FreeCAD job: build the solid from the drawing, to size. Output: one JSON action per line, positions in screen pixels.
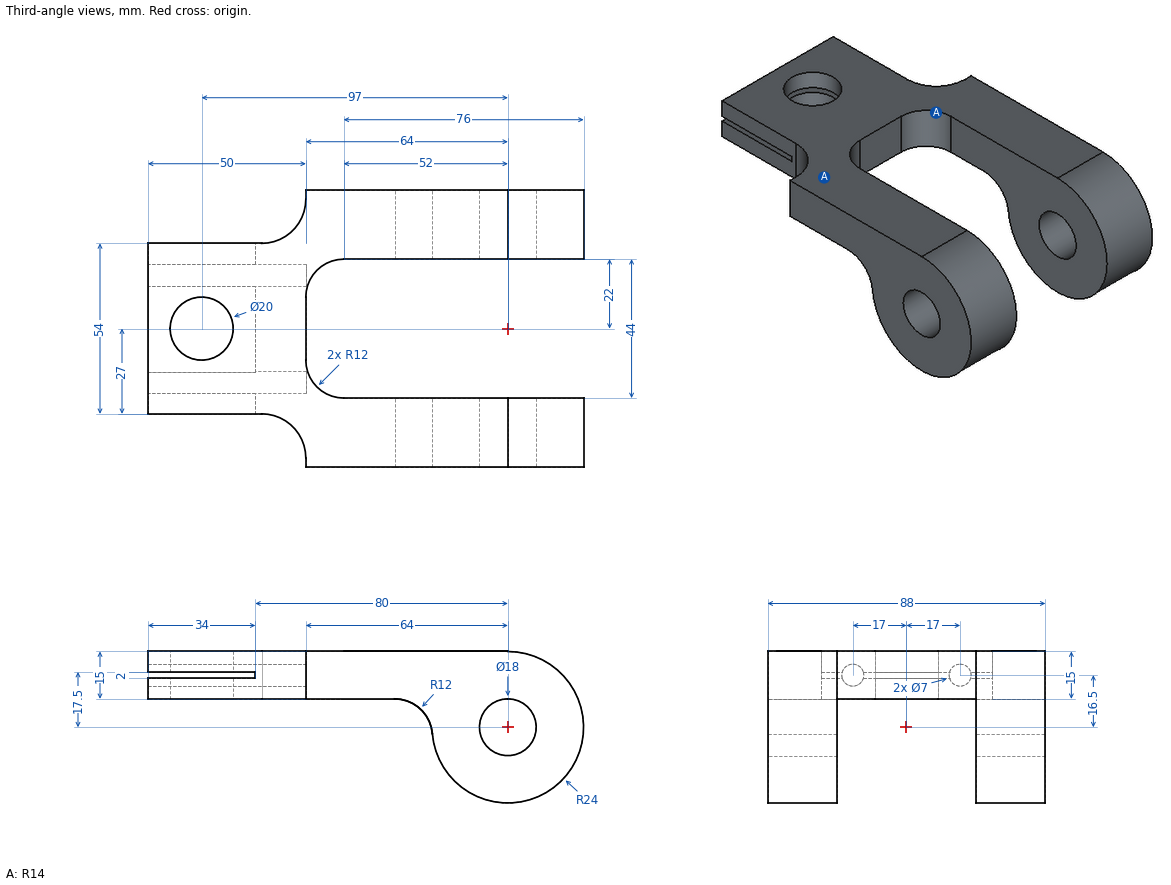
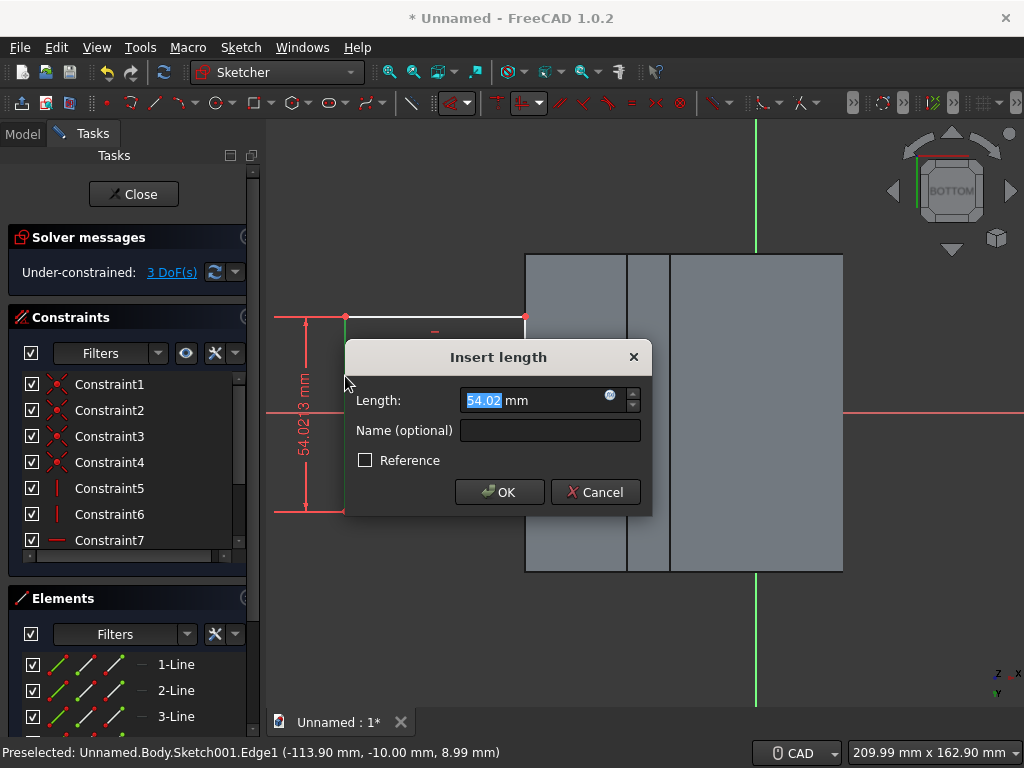
{"action": "type", "text": "54"}
{"action": "key", "text": "Return"}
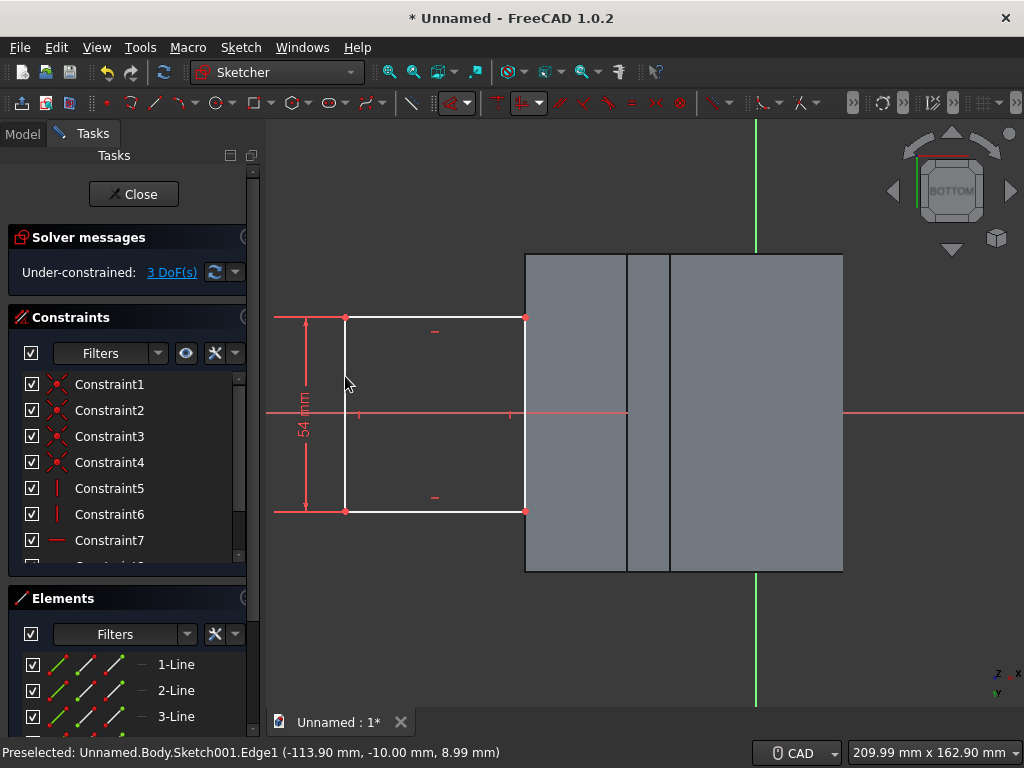
{"action": "left_click", "coordinate": [399, 512]}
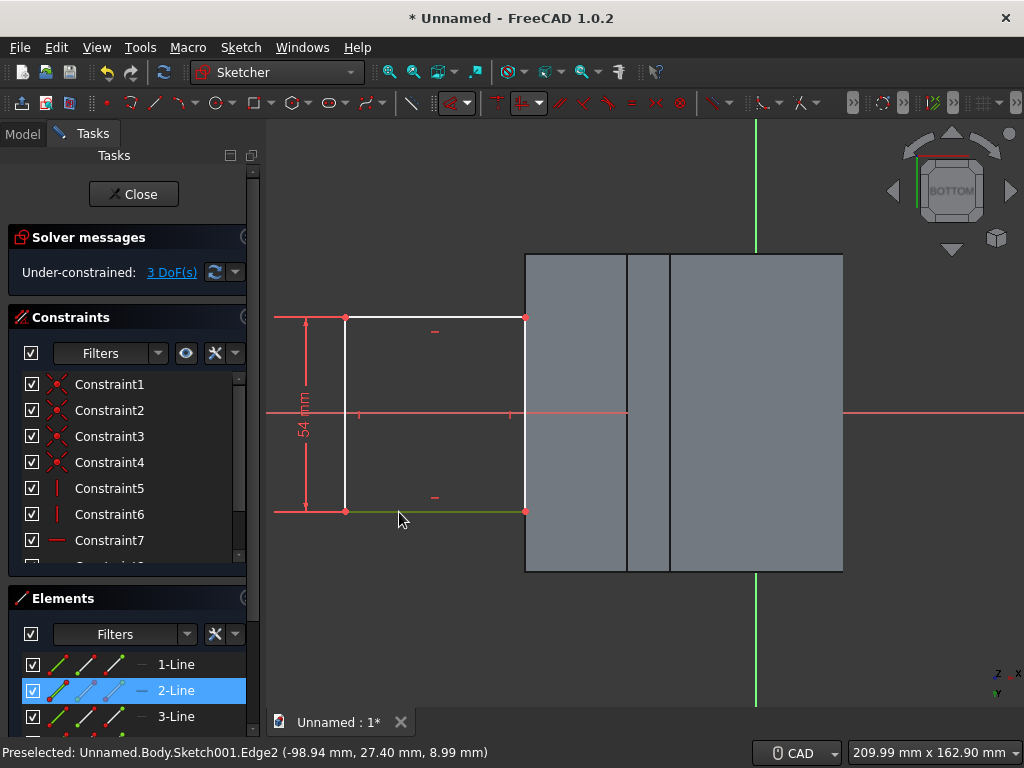
{"action": "key", "text": "l"}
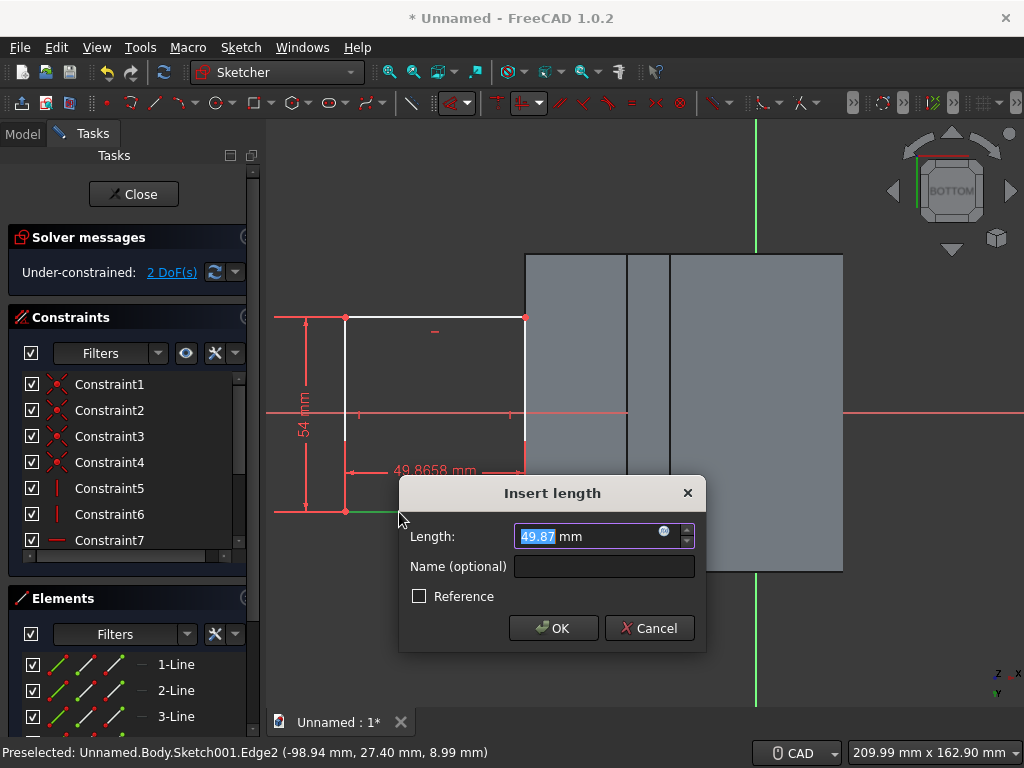
{"action": "type", "text": "50"}
{"action": "key", "text": "Return"}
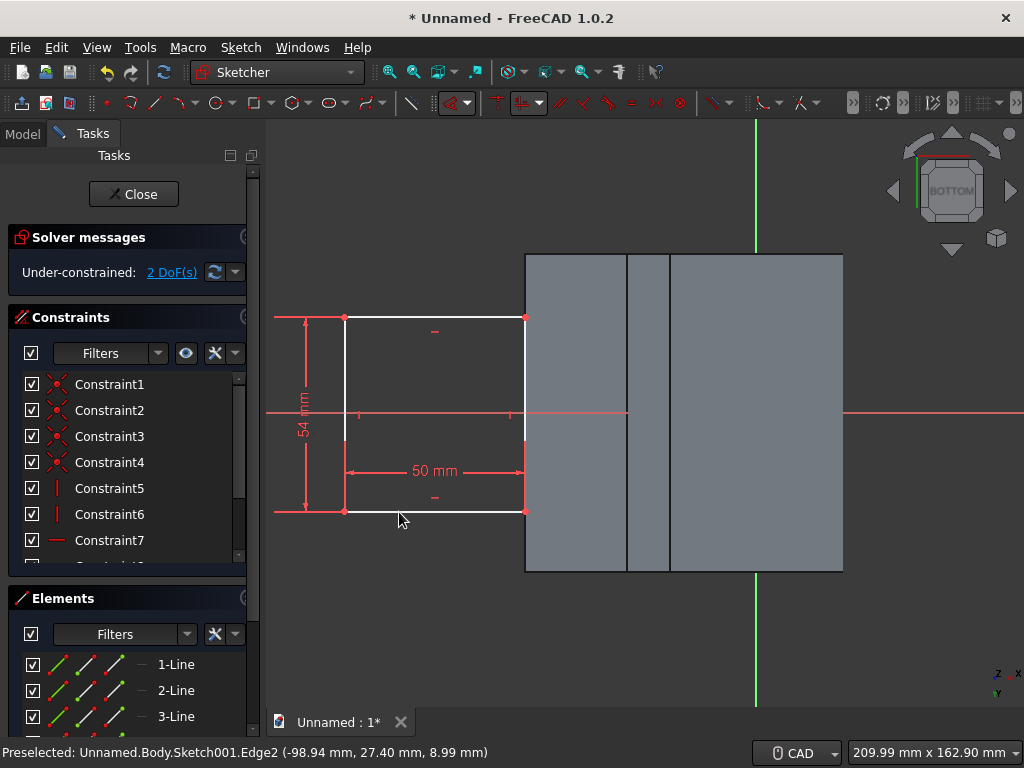
{"action": "left_click", "coordinate": [345, 317]}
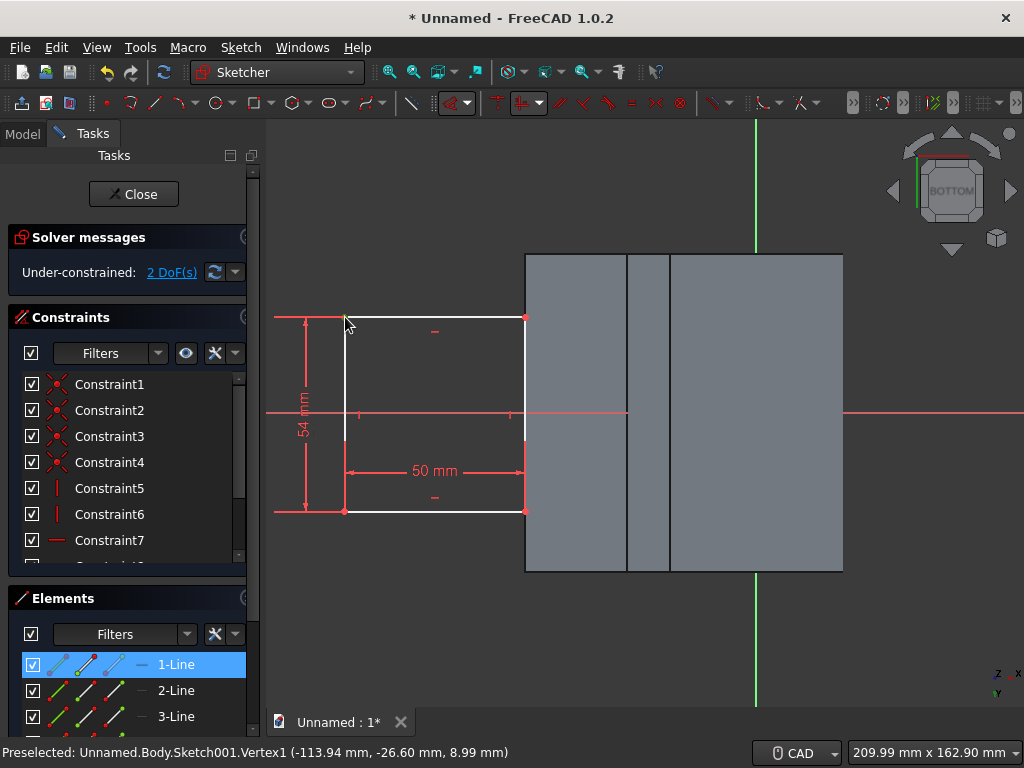
{"action": "key", "text": "i"}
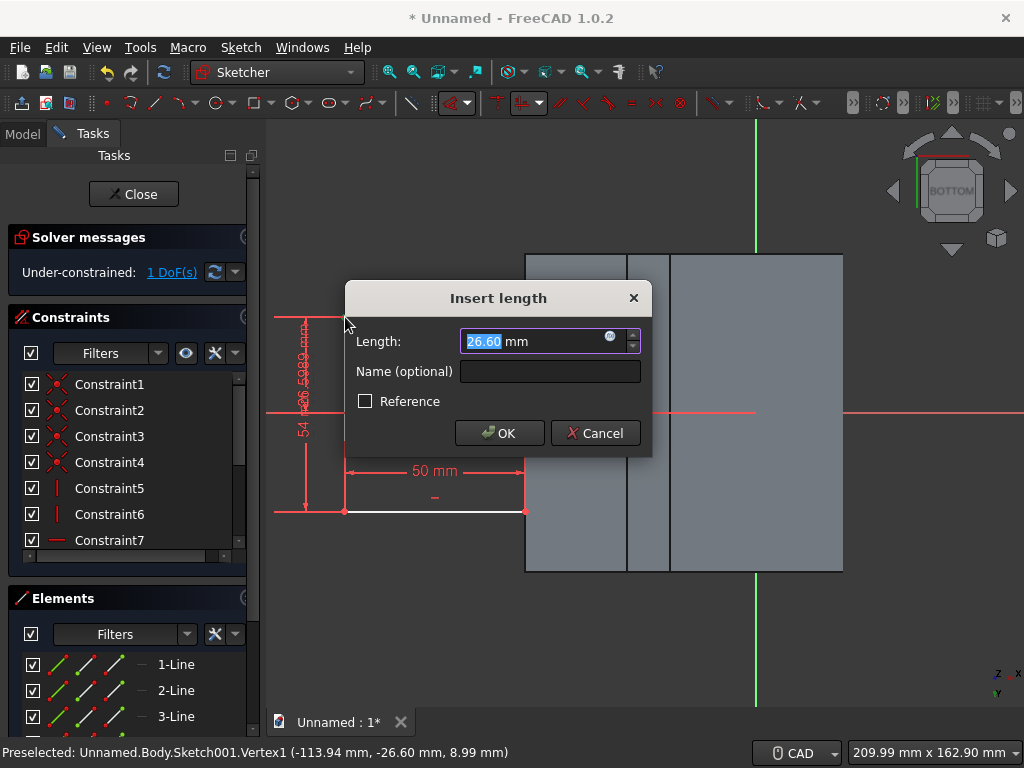
{"action": "type", "text": "27"}
{"action": "key", "text": "Return"}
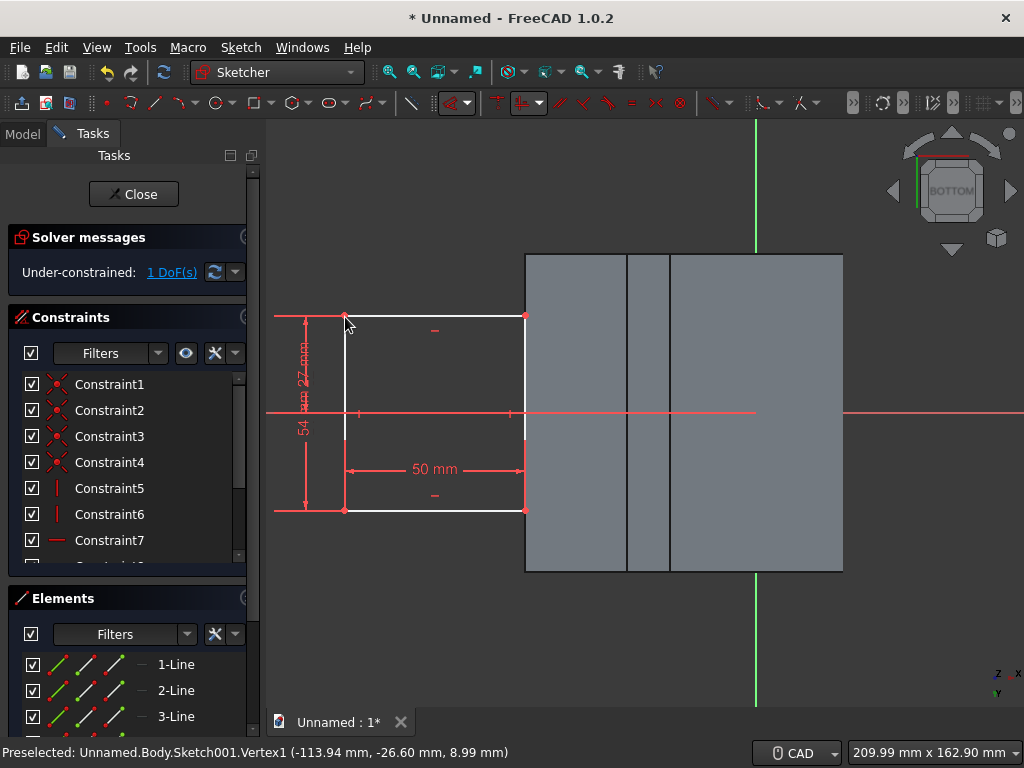
{"action": "left_click", "coordinate": [525, 511]}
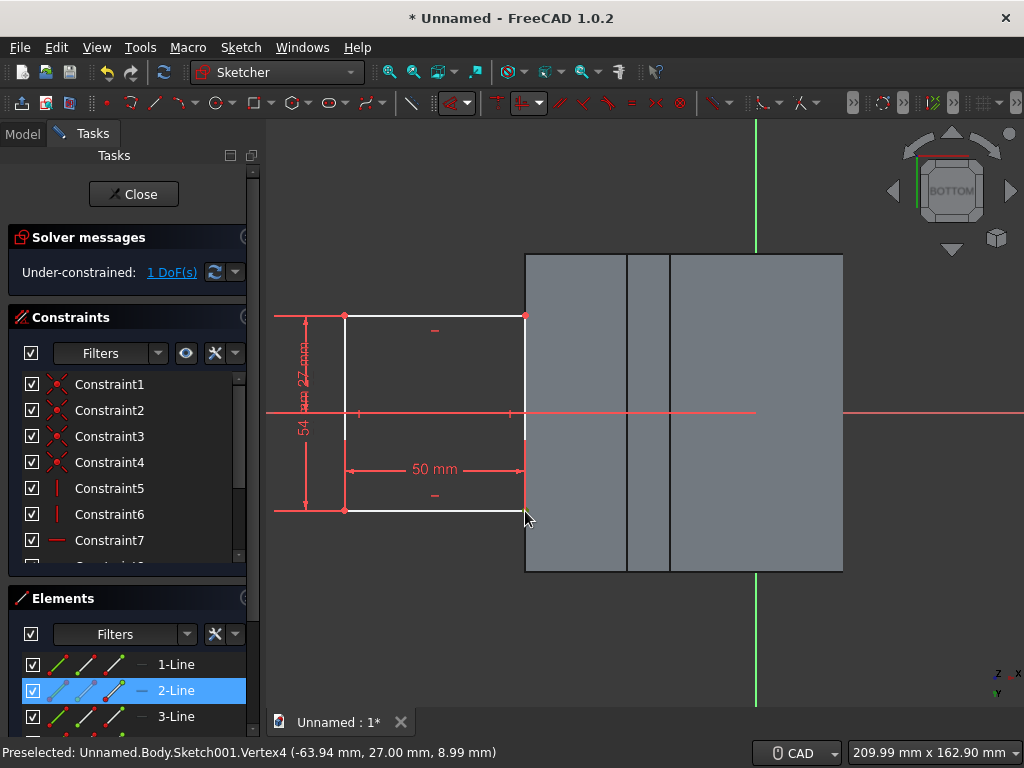
{"action": "key", "text": "l"}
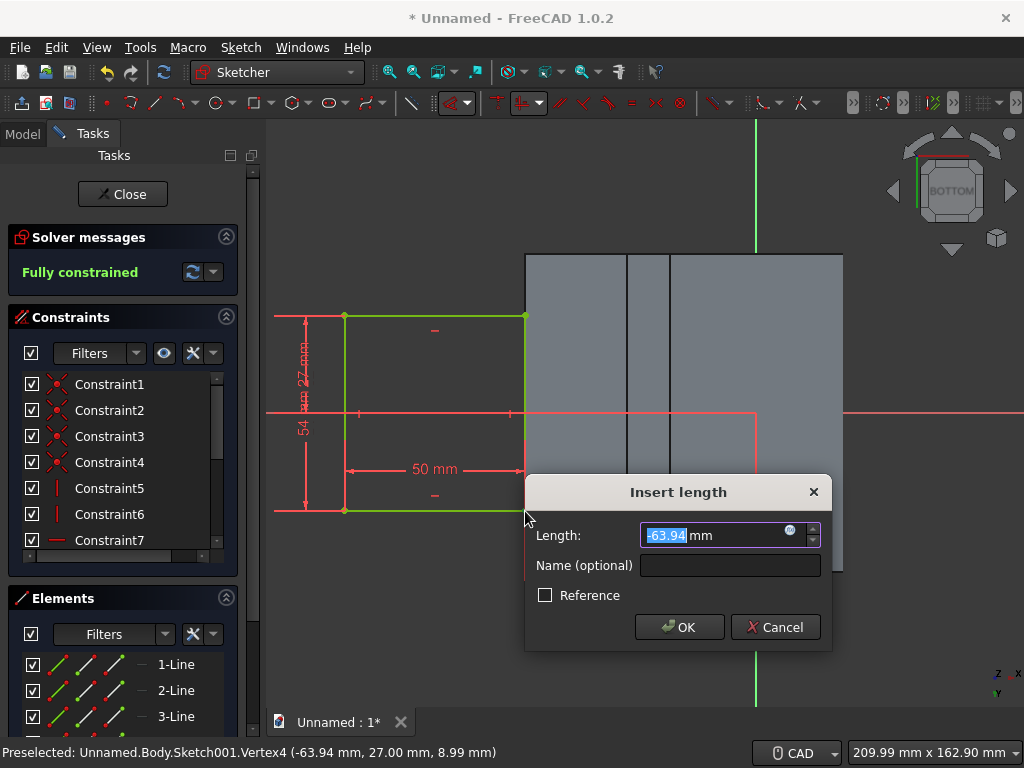
{"action": "type", "text": "-64"}
{"action": "key", "text": "Return"}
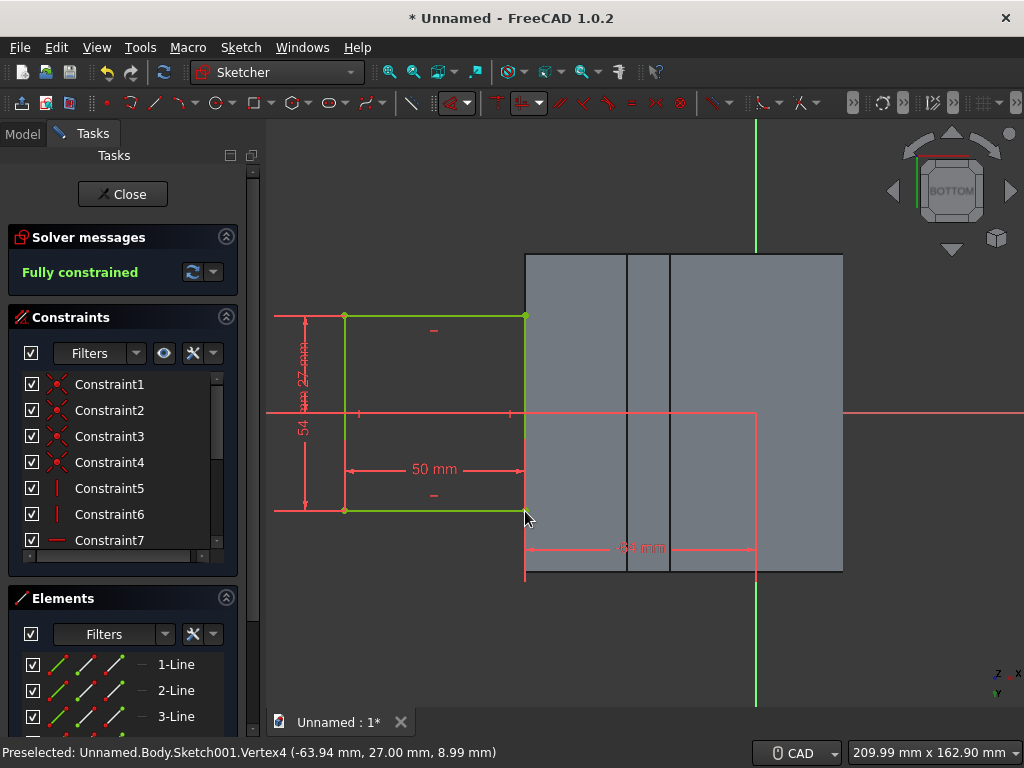
{"action": "left_click", "coordinate": [123, 194]}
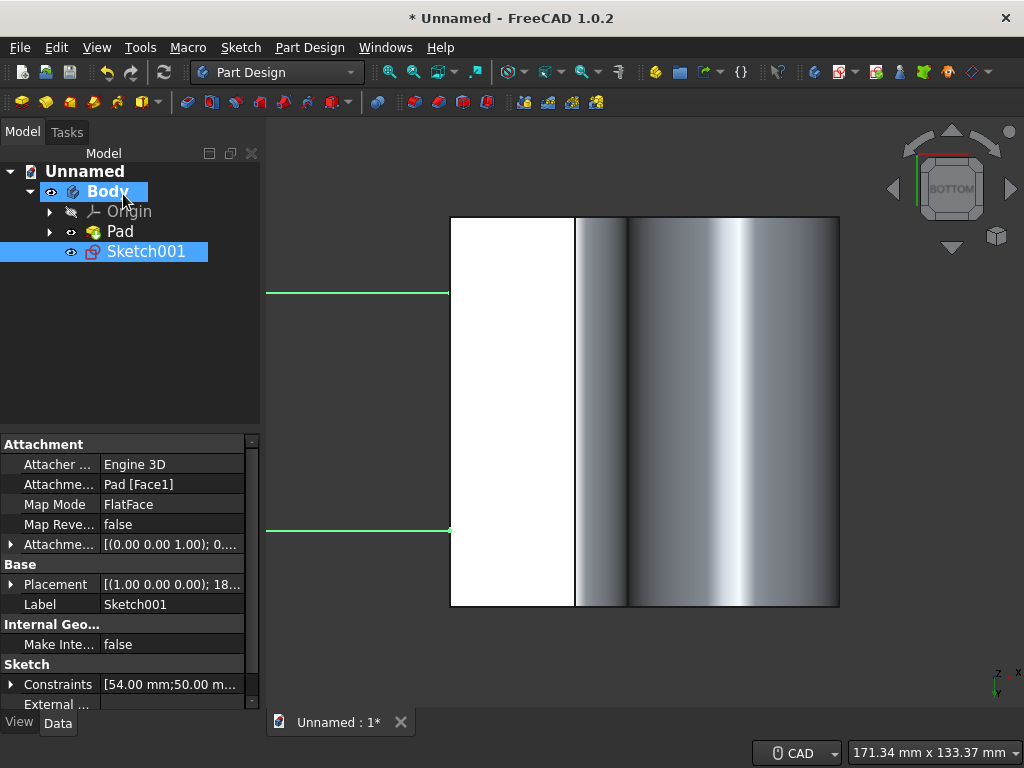
{"action": "left_click", "coordinate": [22, 102]}